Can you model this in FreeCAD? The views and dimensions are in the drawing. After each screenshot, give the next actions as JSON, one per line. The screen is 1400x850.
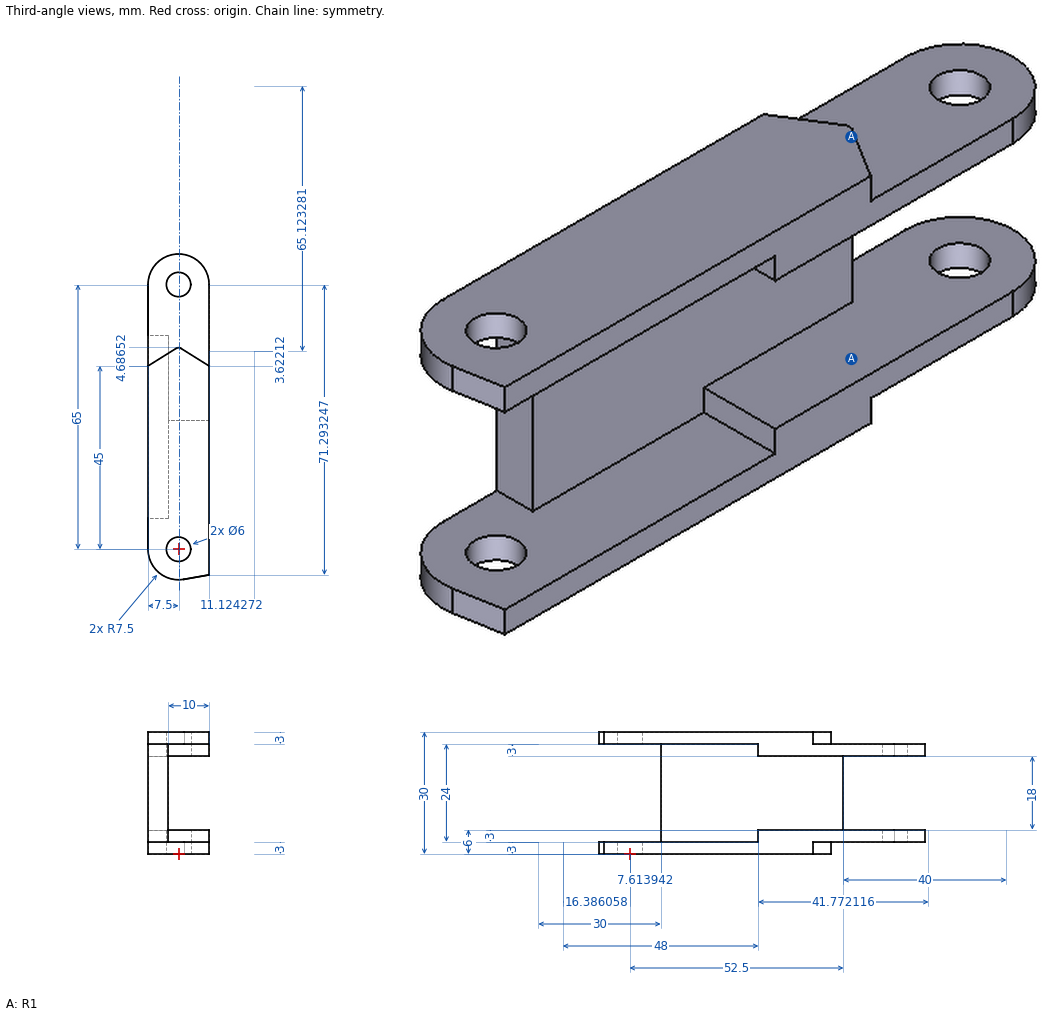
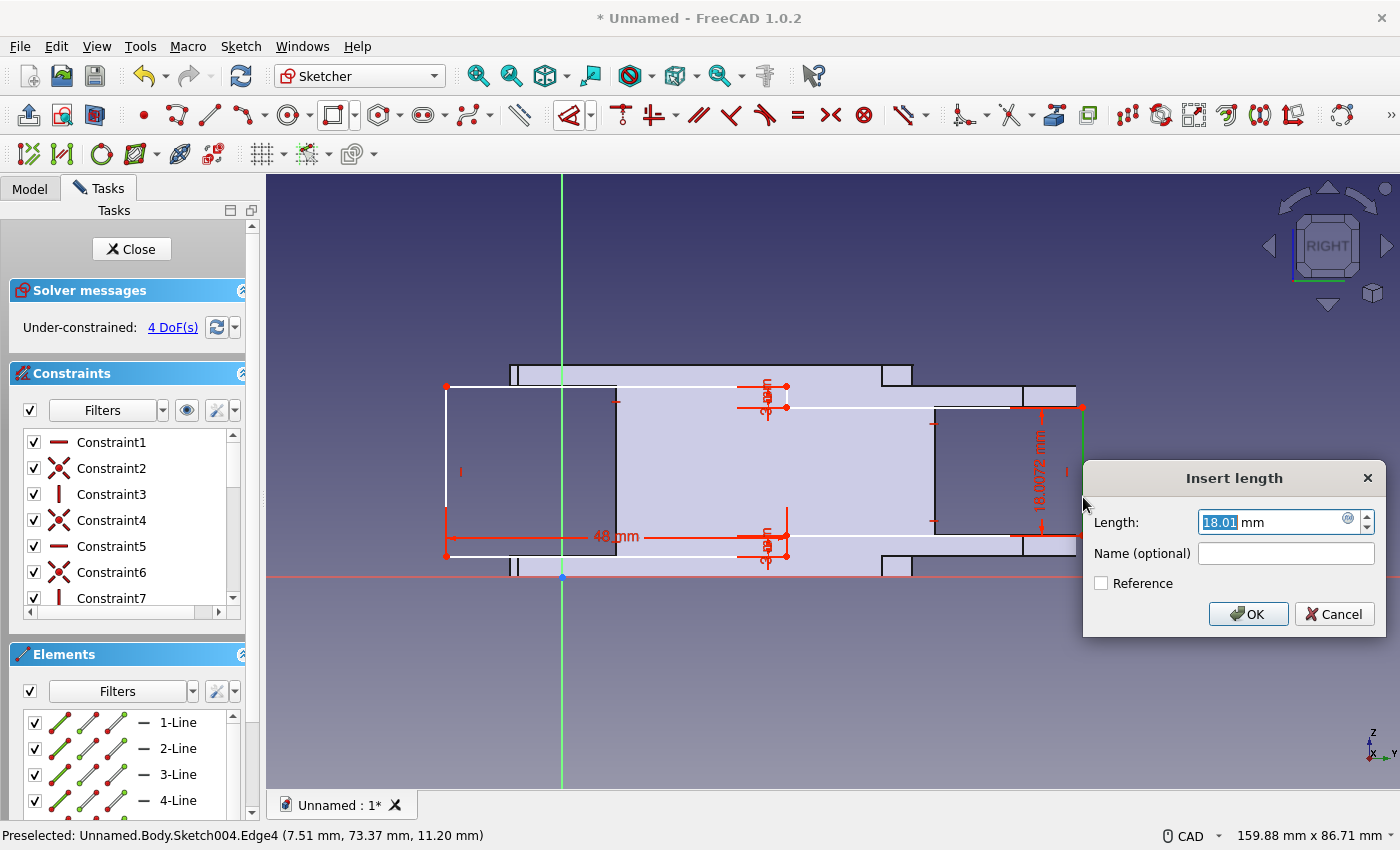
{"action": "type", "text": "18"}
{"action": "key", "text": "Return"}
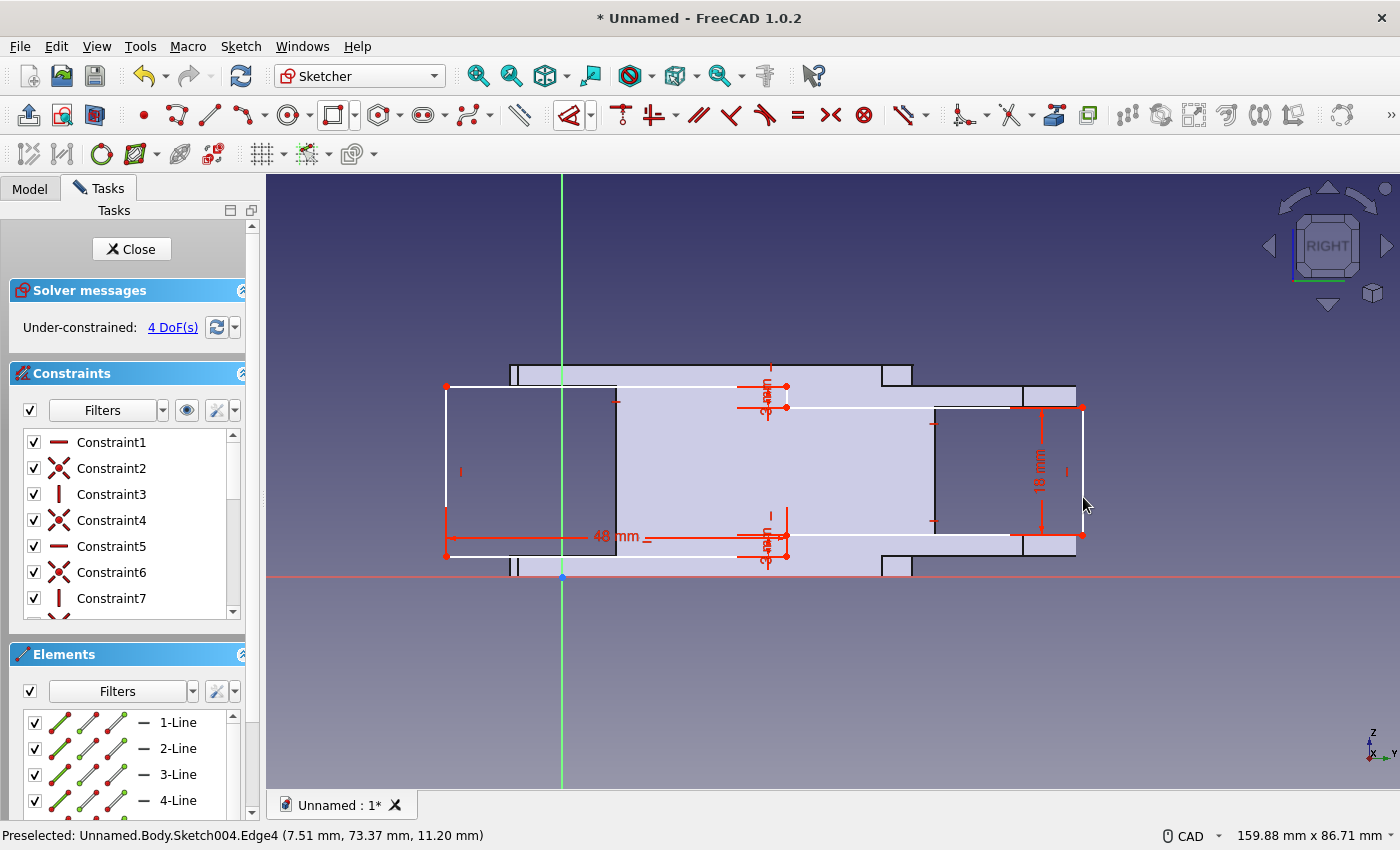
{"action": "left_click", "coordinate": [685, 387]}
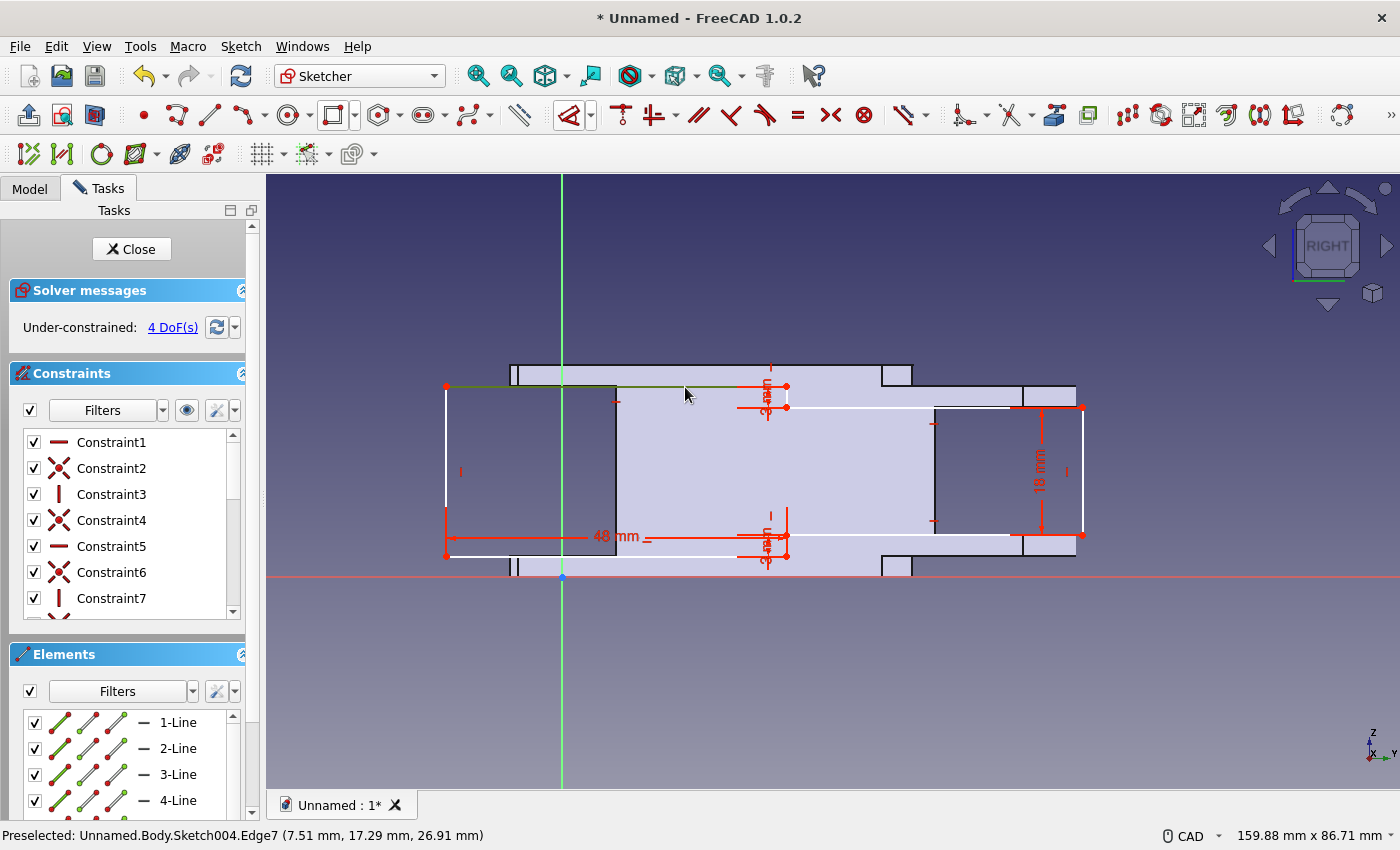
{"action": "key", "text": "l"}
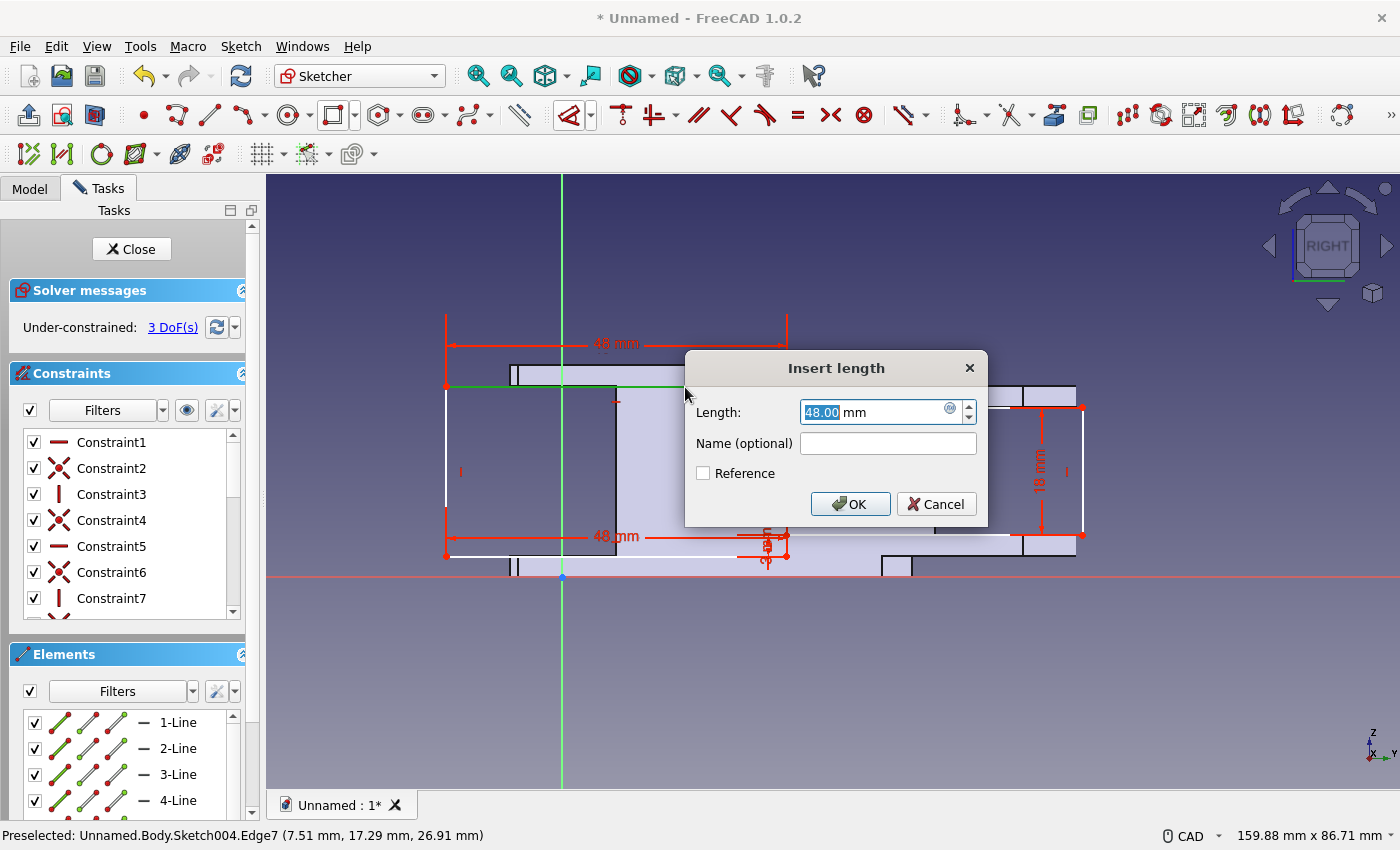
{"action": "type", "text": "48"}
{"action": "key", "text": "Return"}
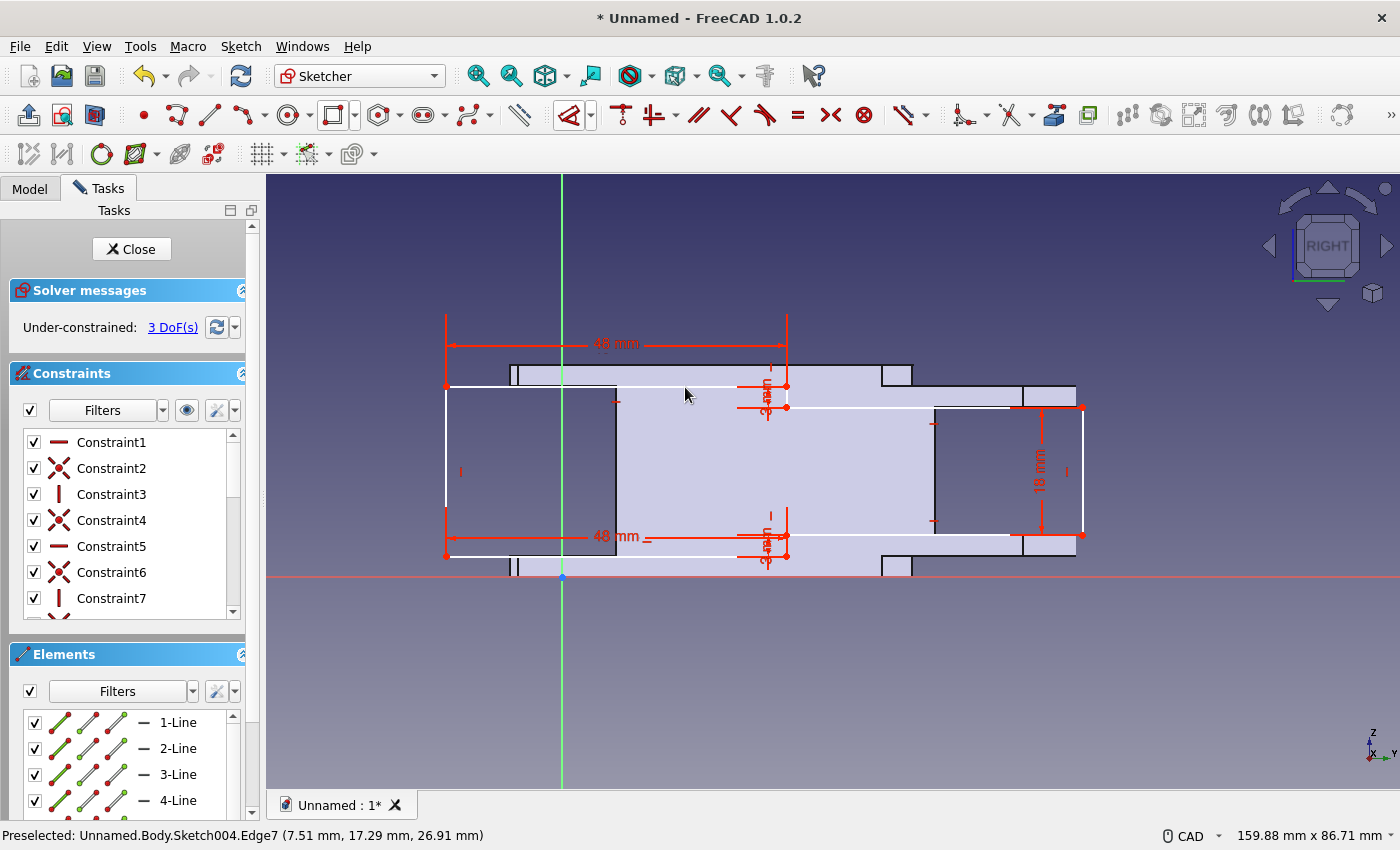
{"action": "scroll", "coordinate": [446, 557], "scroll_direction": "up", "scroll_amount": 4}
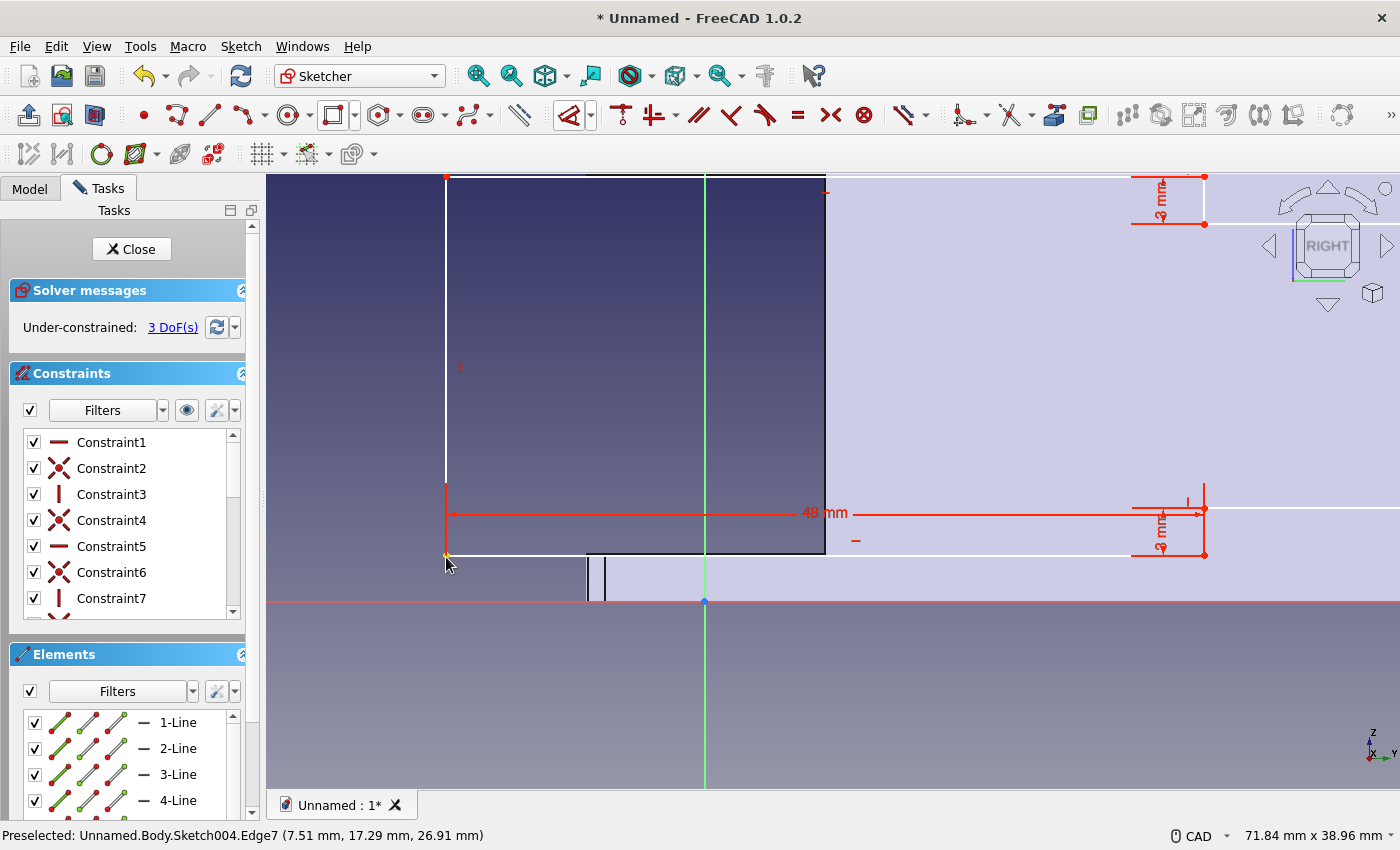
{"action": "left_click", "coordinate": [446, 556]}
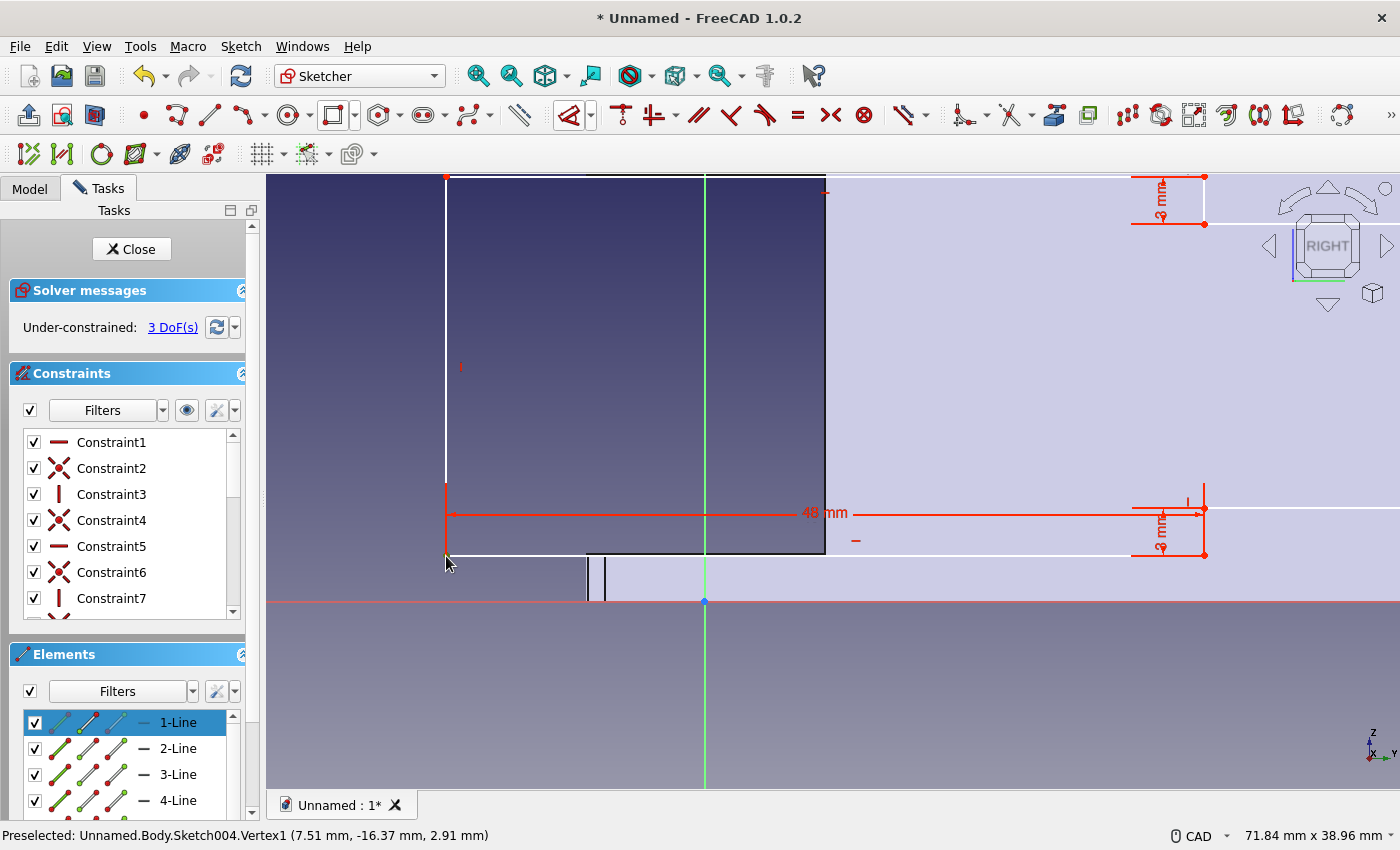
{"action": "left_click", "coordinate": [590, 116]}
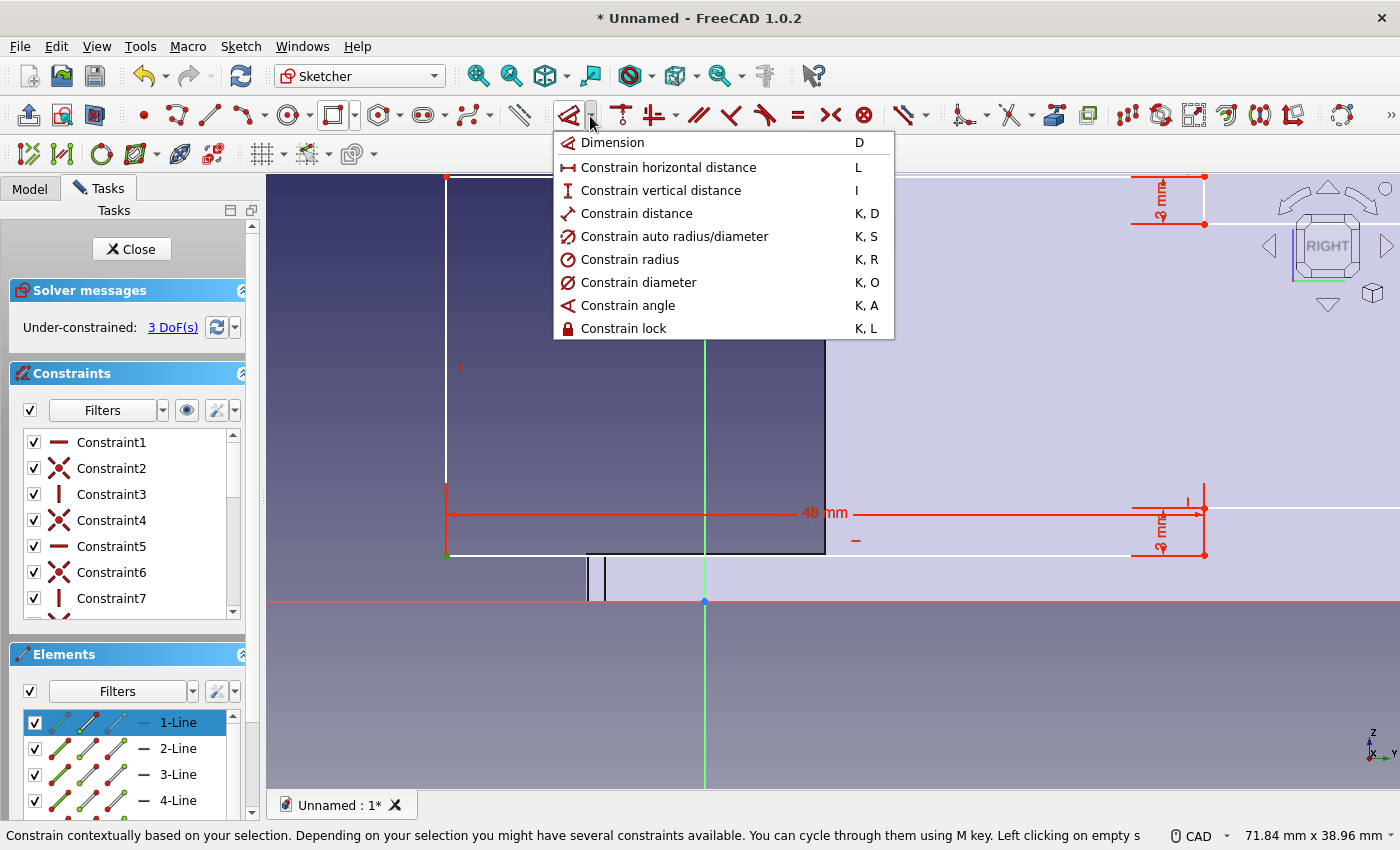
{"action": "left_click", "coordinate": [724, 190]}